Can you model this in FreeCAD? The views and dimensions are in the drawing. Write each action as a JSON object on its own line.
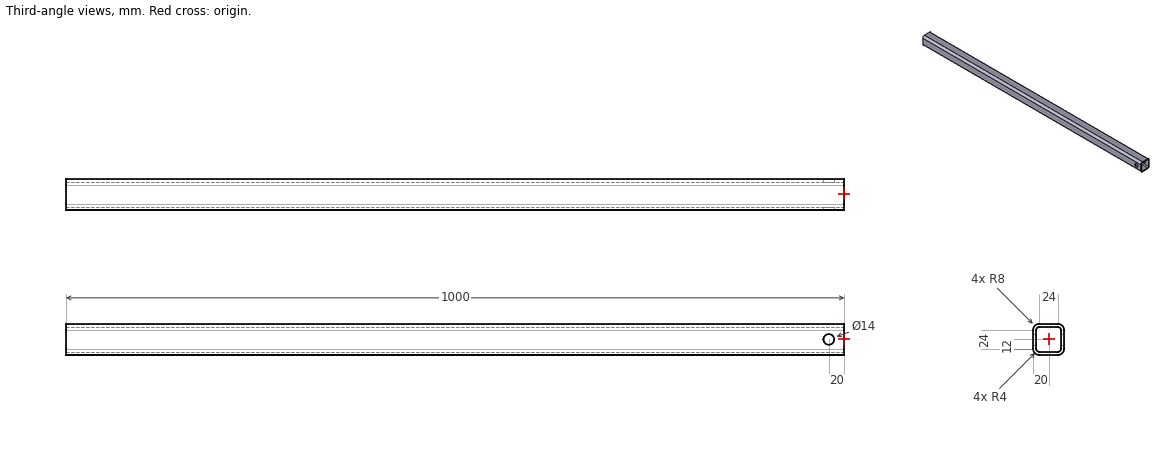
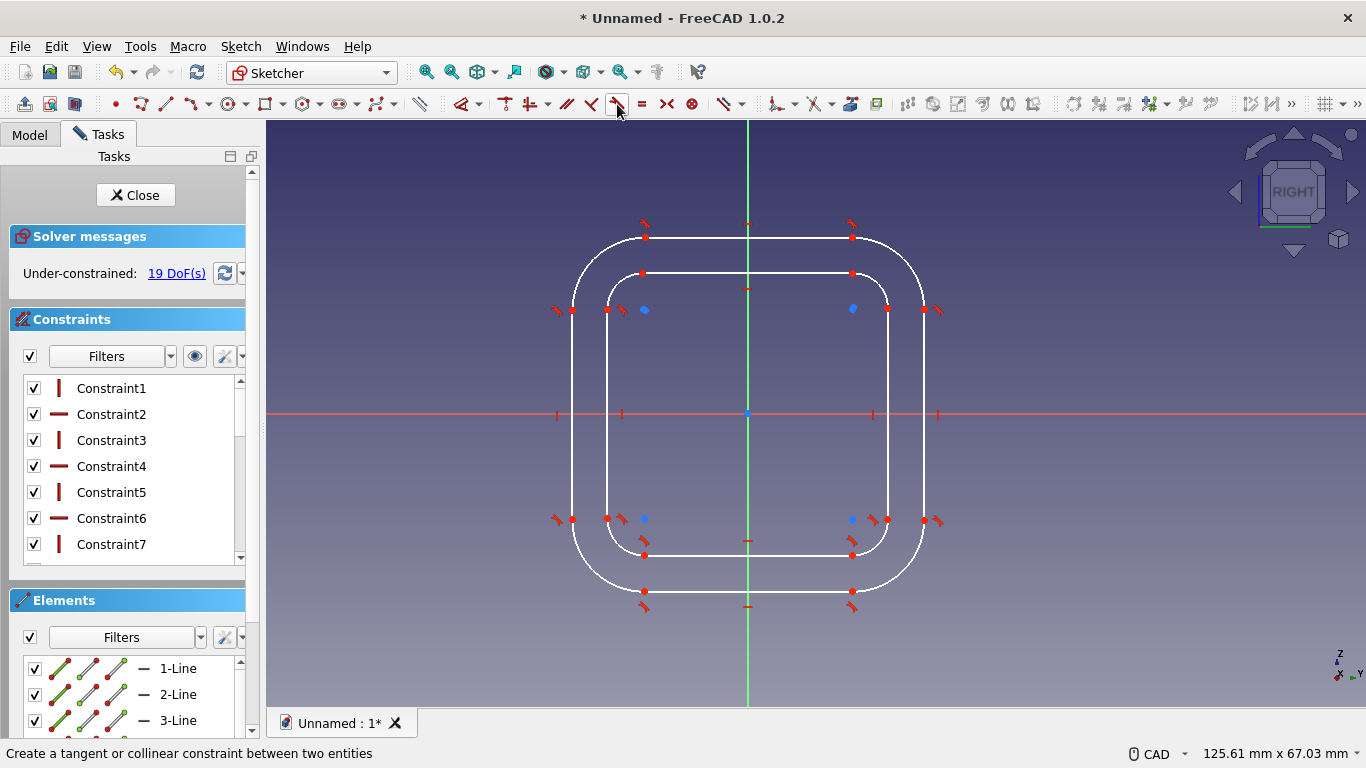
{"action": "left_click", "coordinate": [888, 457]}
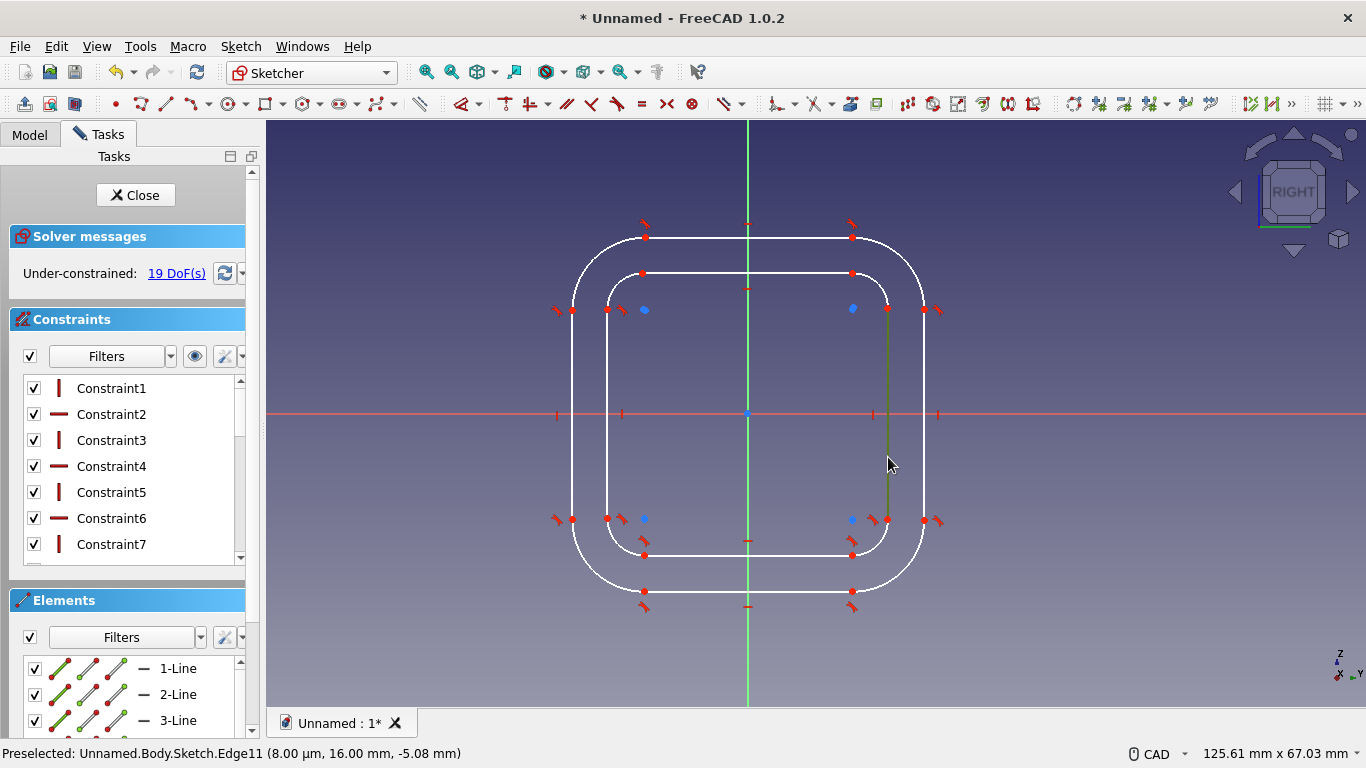
{"action": "left_click", "coordinate": [884, 293]}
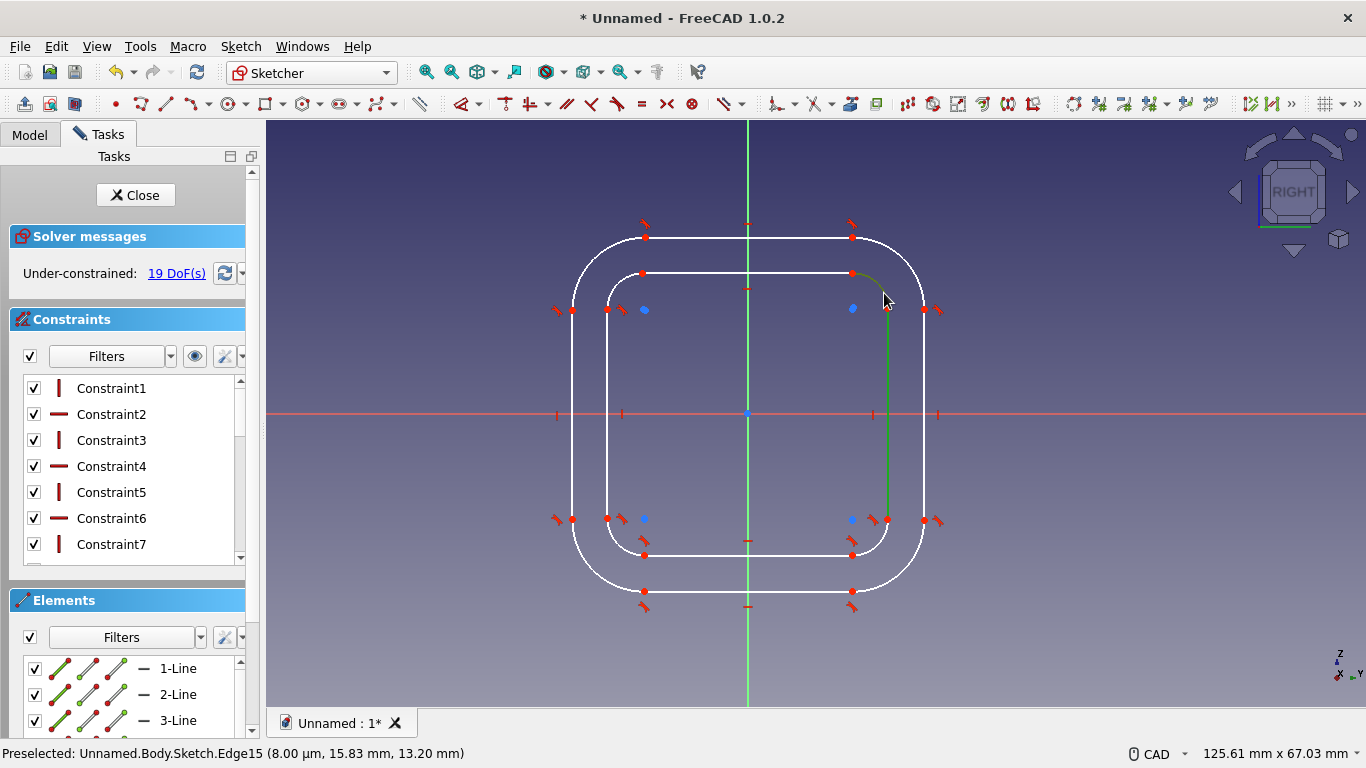
{"action": "left_click", "coordinate": [617, 104]}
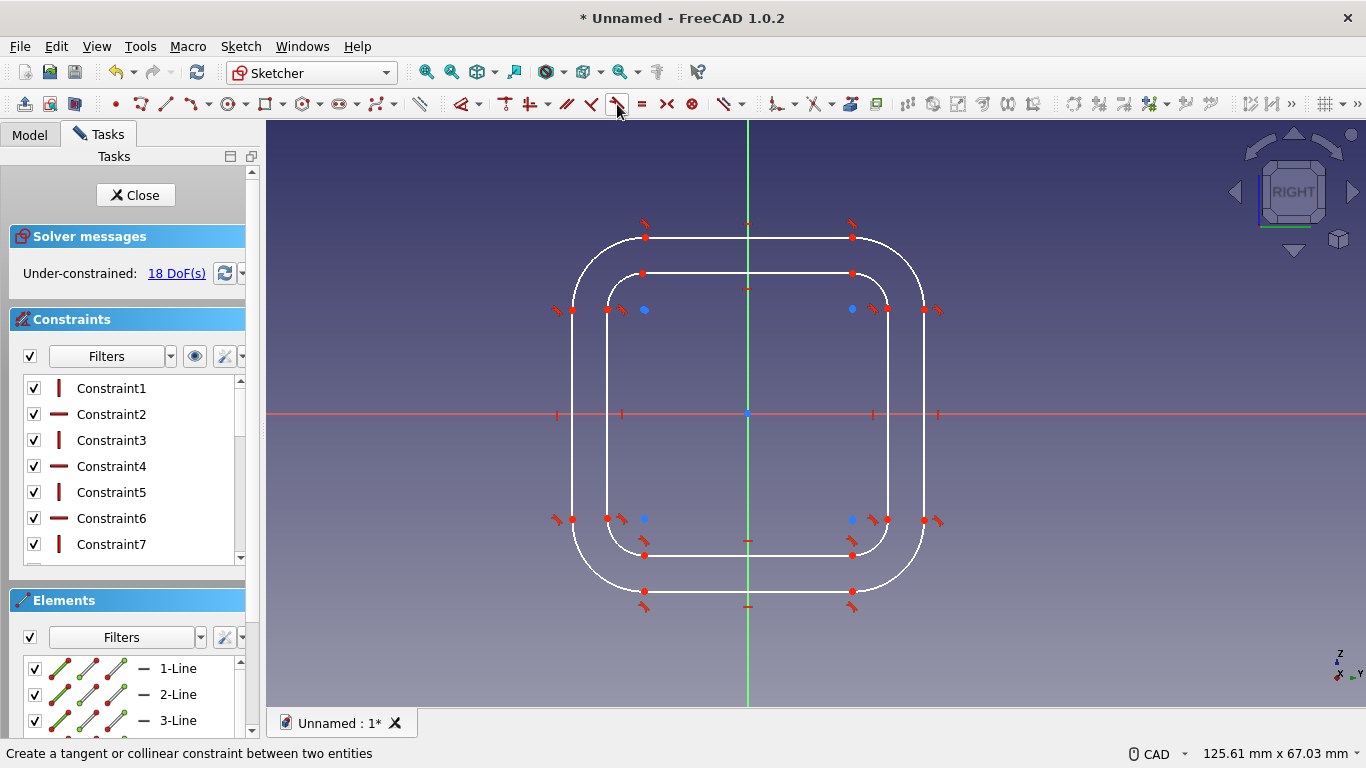
{"action": "left_click", "coordinate": [789, 273]}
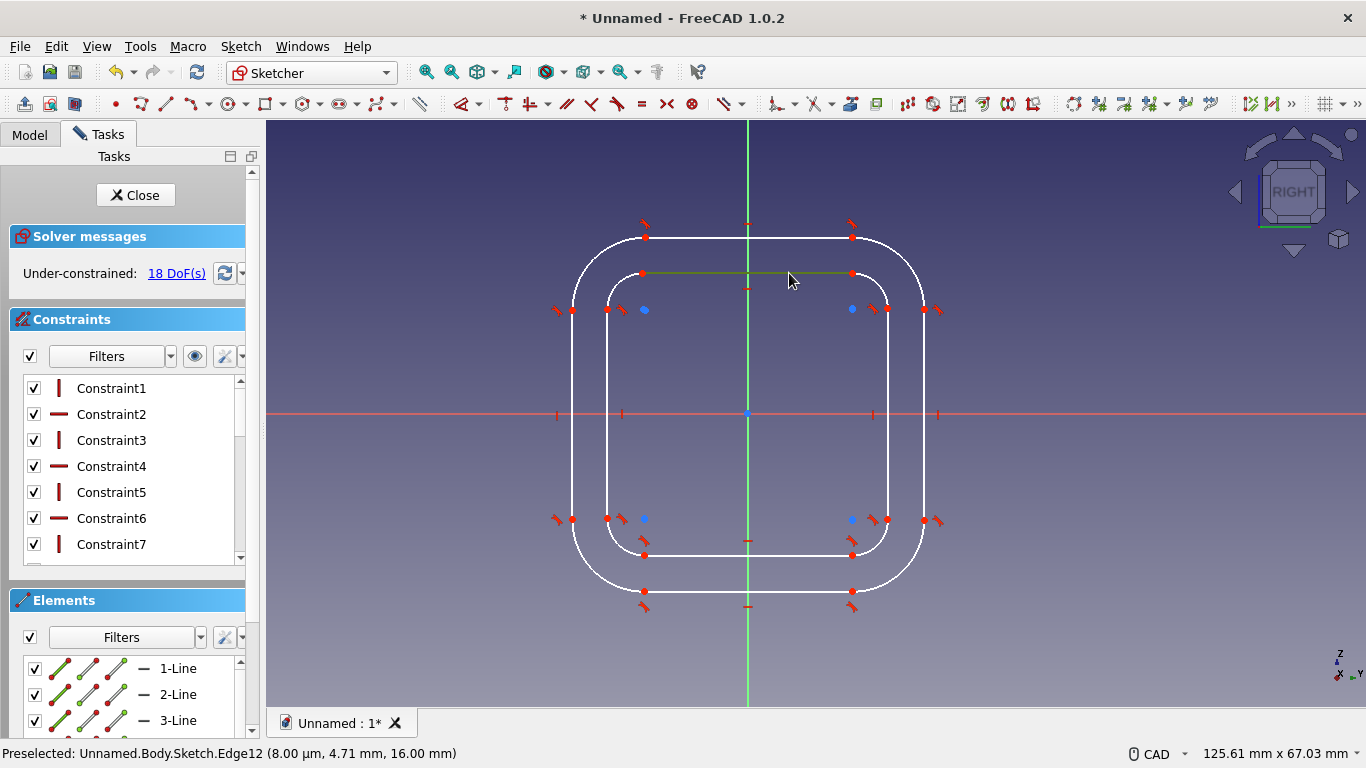
{"action": "left_click", "coordinate": [884, 293]}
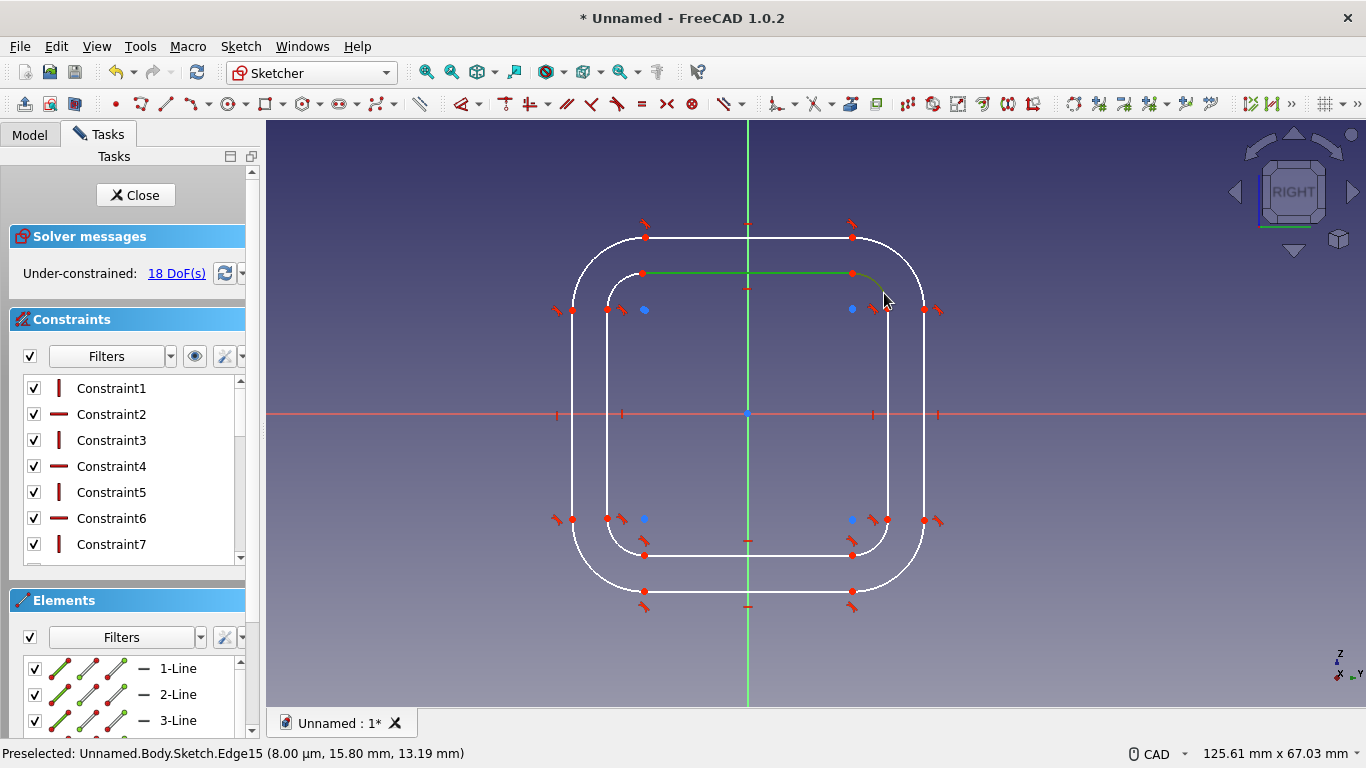
{"action": "left_click", "coordinate": [617, 104]}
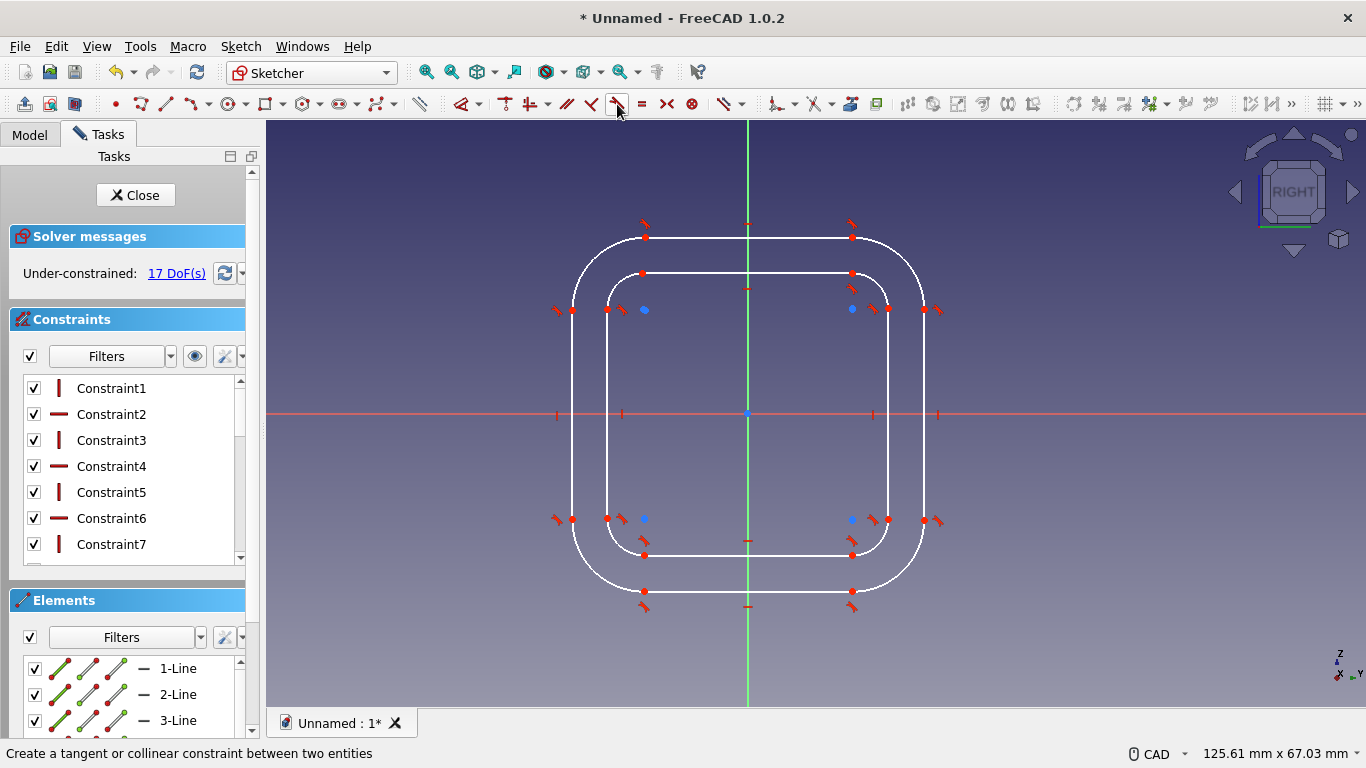
{"action": "left_click", "coordinate": [789, 273]}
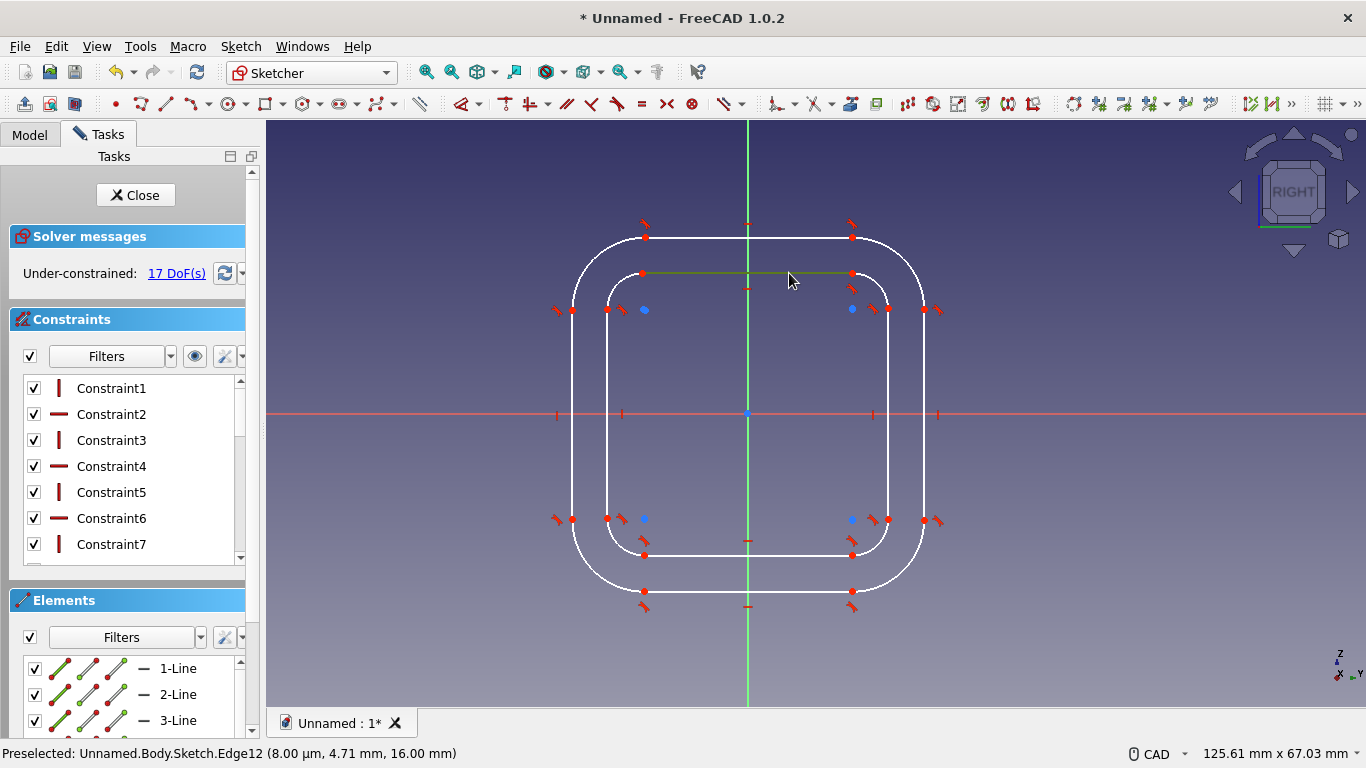
{"action": "left_click", "coordinate": [627, 277]}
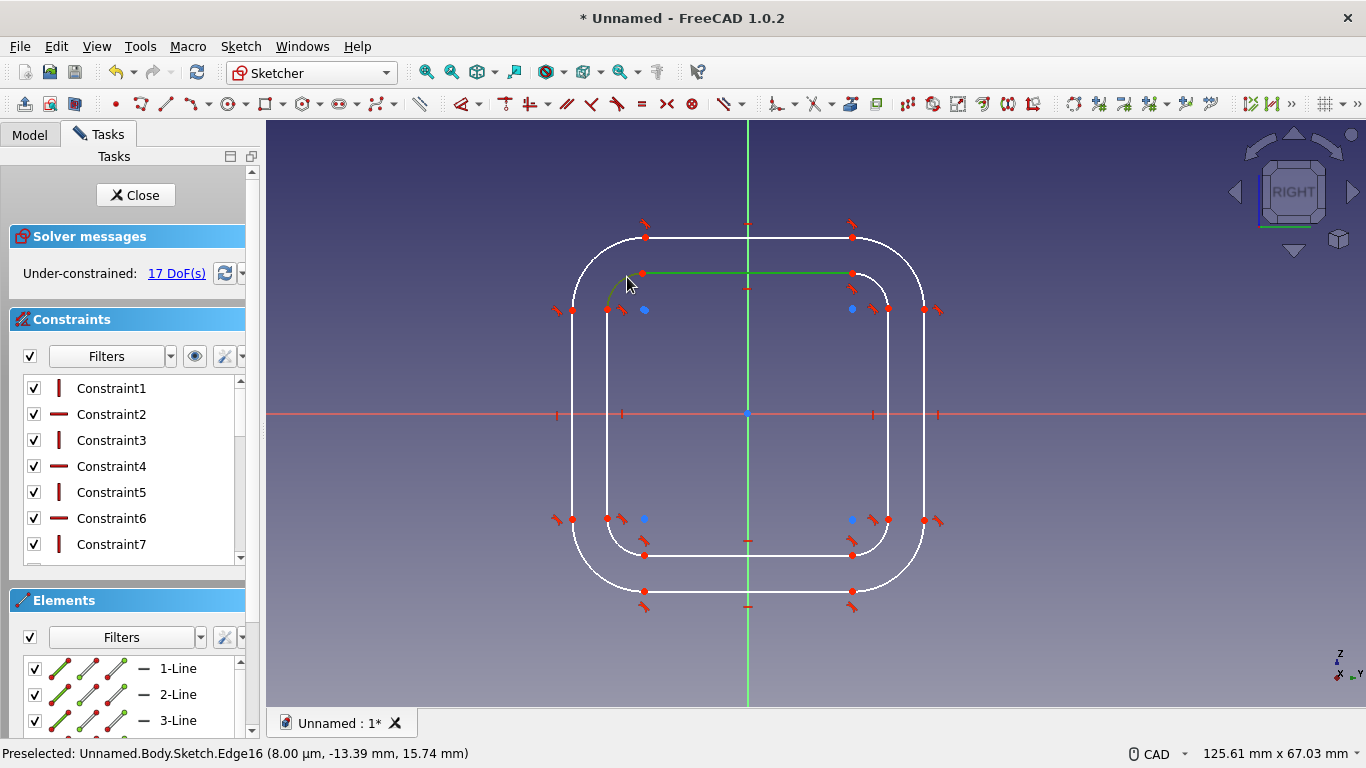
{"action": "left_click", "coordinate": [617, 104]}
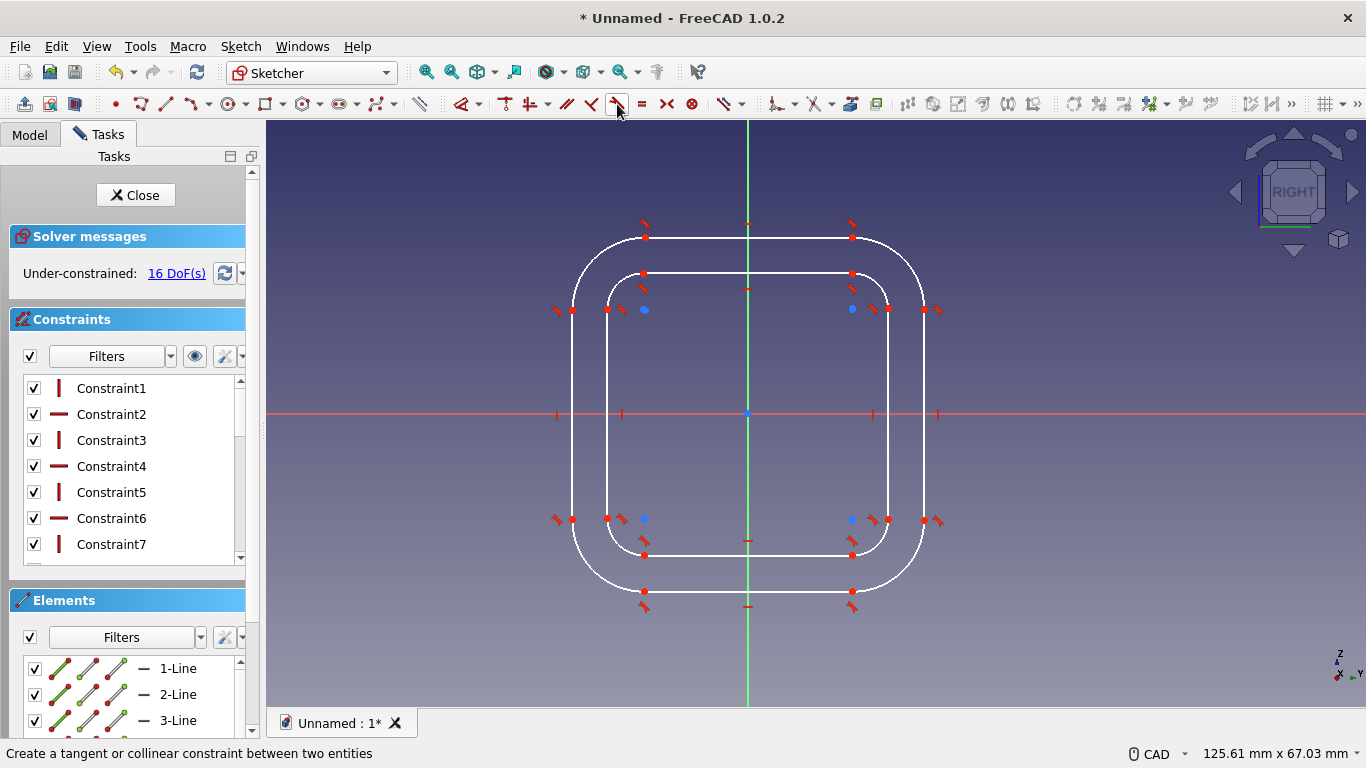
{"action": "left_click", "coordinate": [580, 553]}